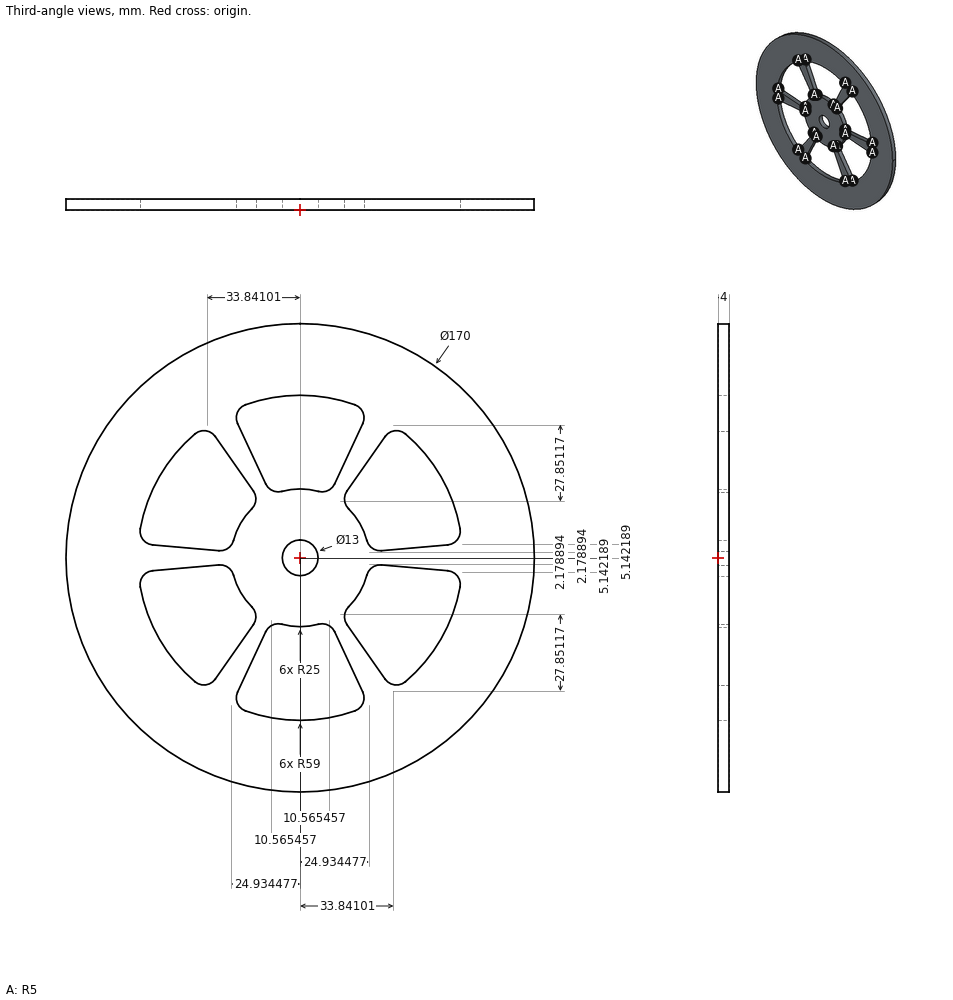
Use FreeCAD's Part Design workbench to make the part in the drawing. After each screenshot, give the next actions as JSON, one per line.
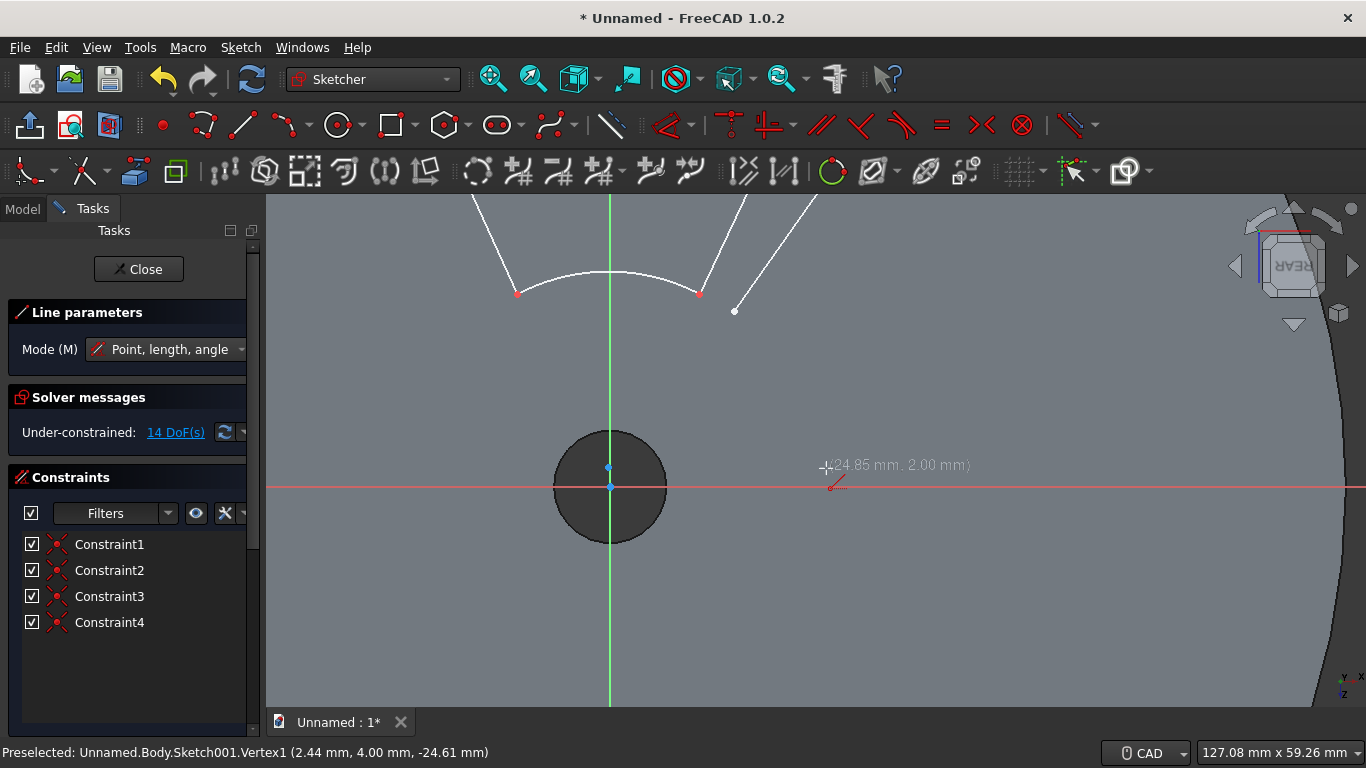
{"action": "left_click", "coordinate": [826, 468]}
{"action": "left_click", "coordinate": [1119, 442]}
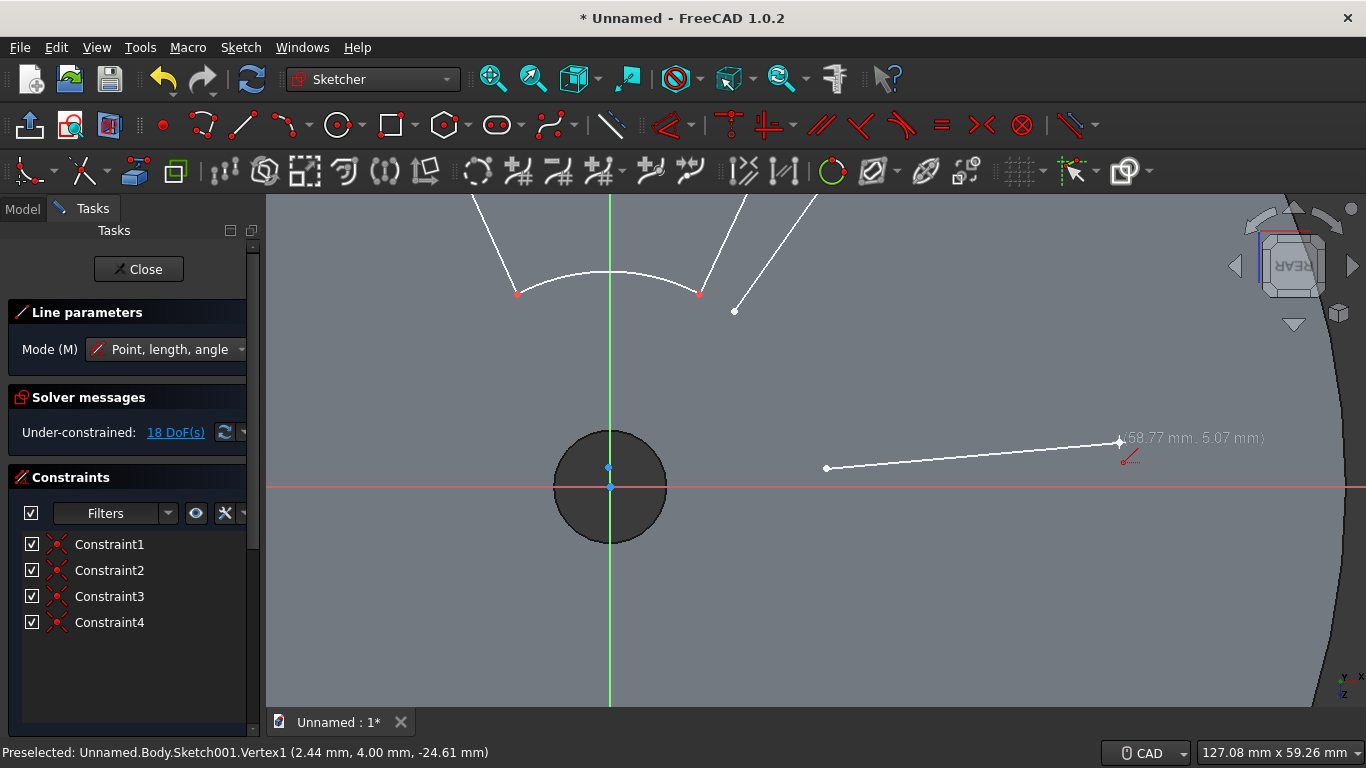
{"action": "left_click", "coordinate": [284, 126]}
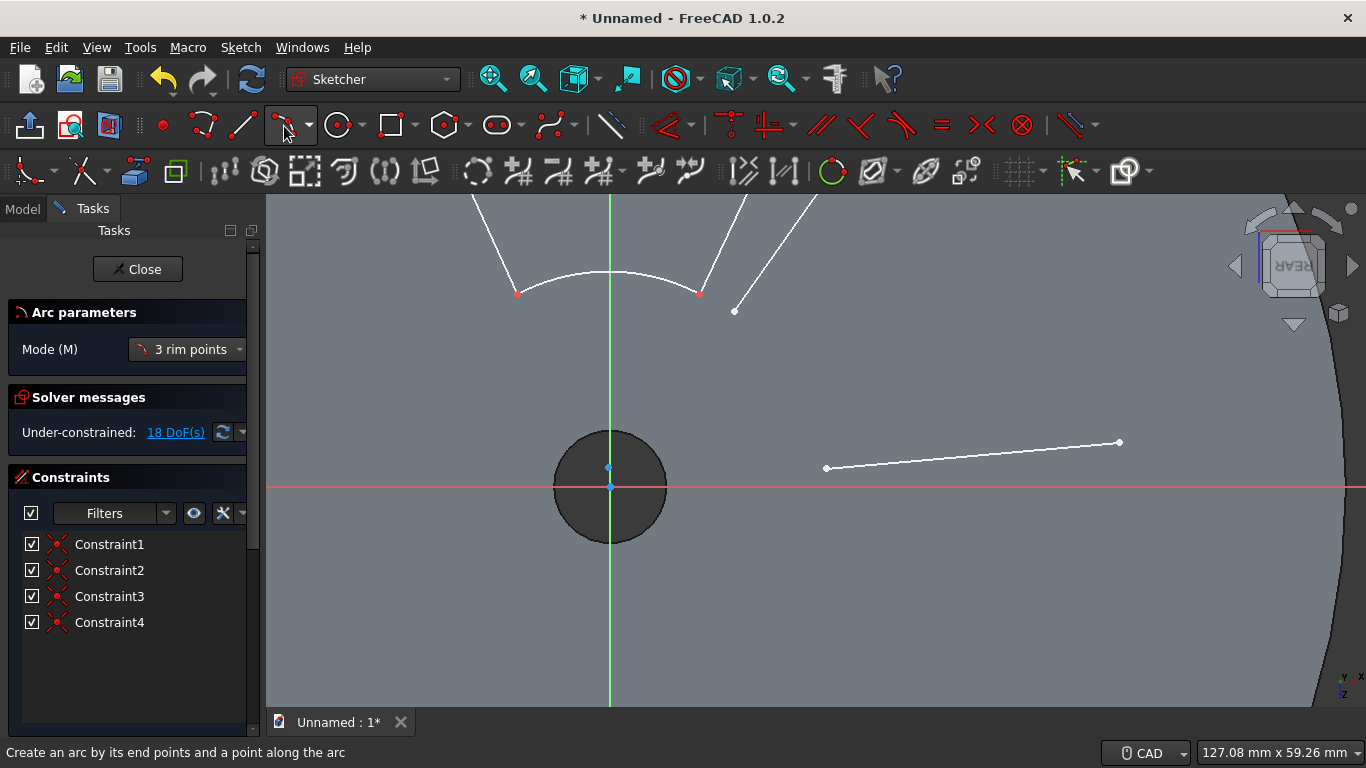
{"action": "left_click", "coordinate": [734, 312]}
{"action": "left_click", "coordinate": [826, 469]}
{"action": "left_click", "coordinate": [798, 379]}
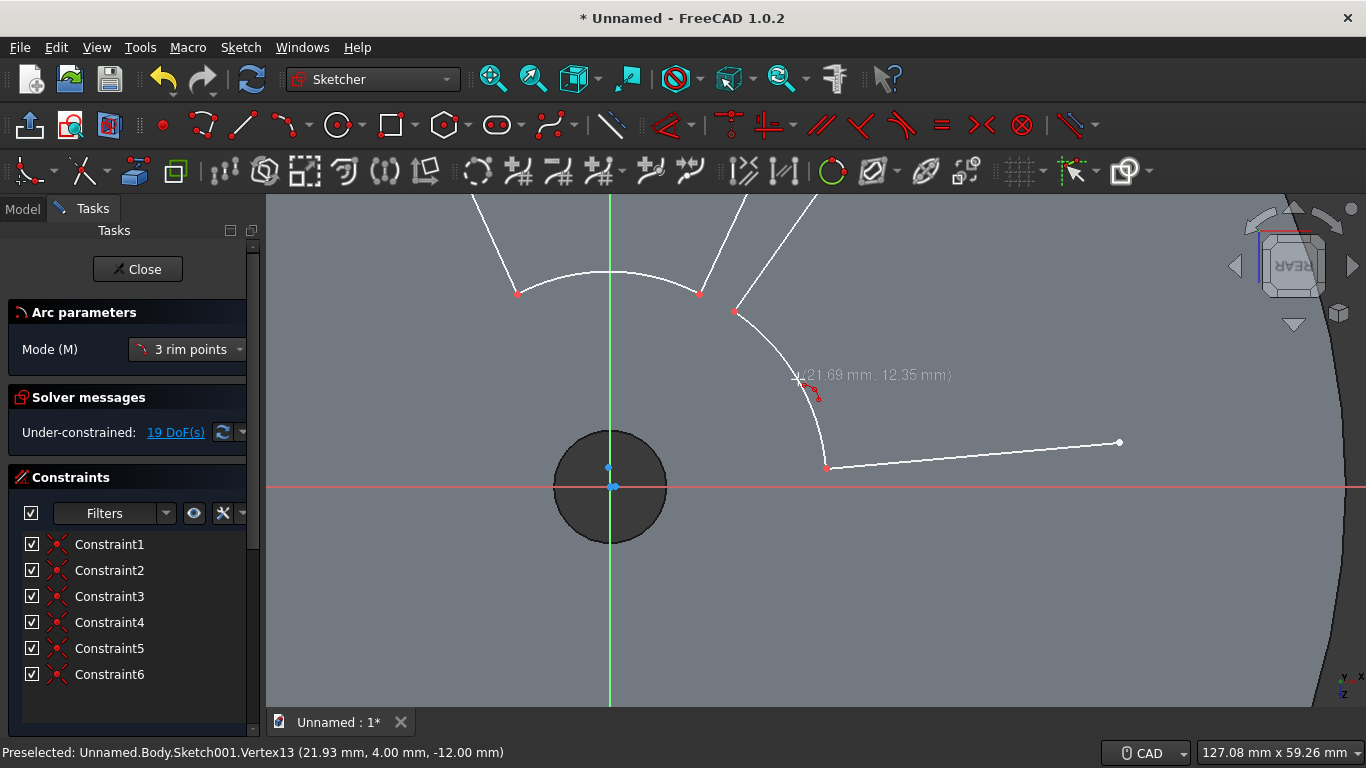
{"action": "left_click", "coordinate": [1119, 443]}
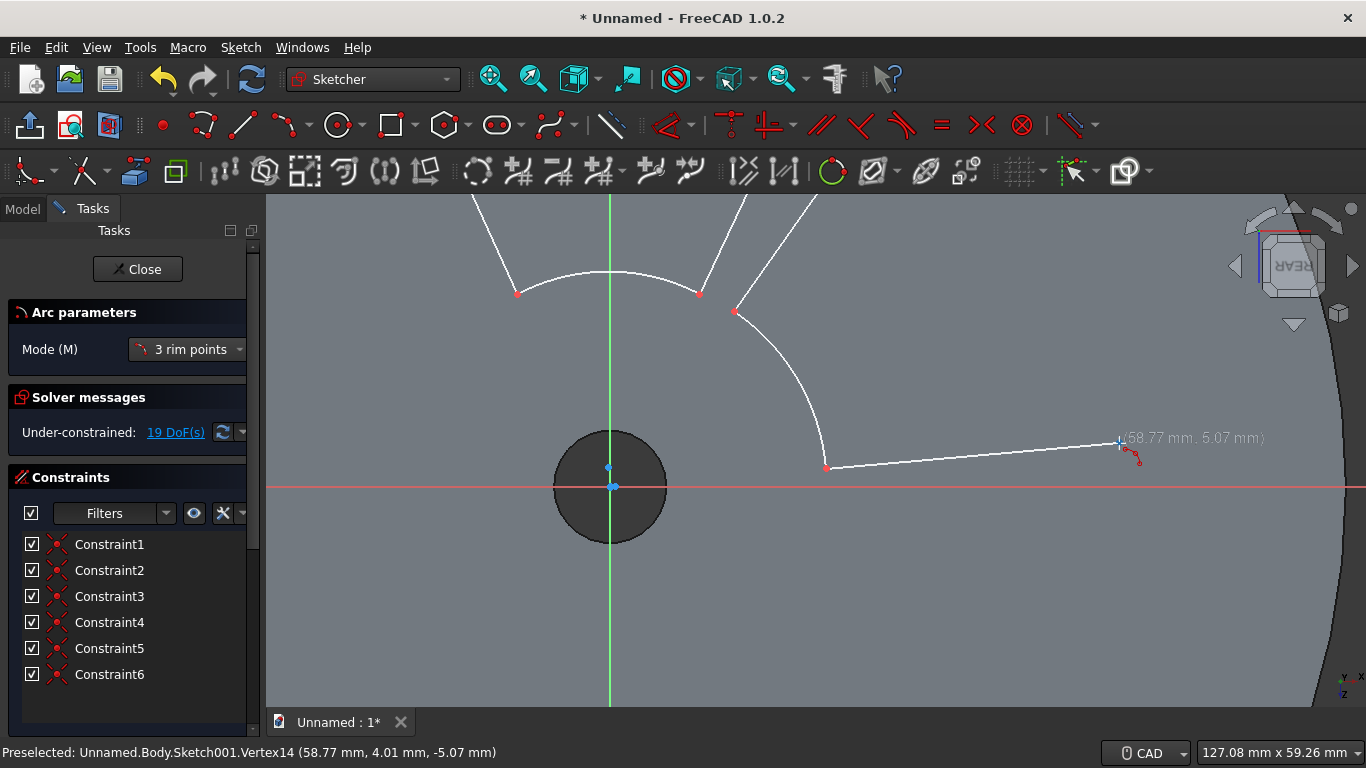
{"action": "scroll", "coordinate": [807, 435], "scroll_direction": "down", "scroll_amount": 6}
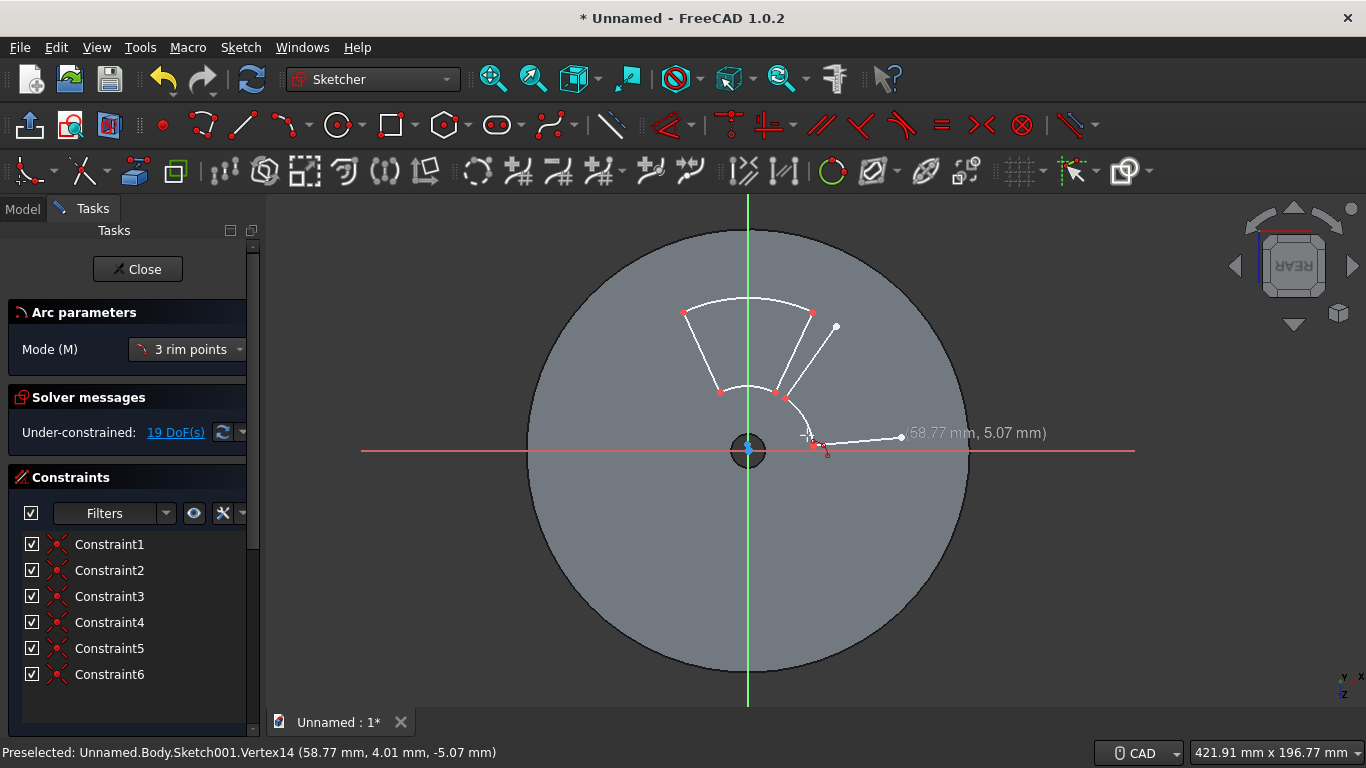
{"action": "left_click", "coordinate": [836, 326]}
{"action": "left_click", "coordinate": [881, 374]}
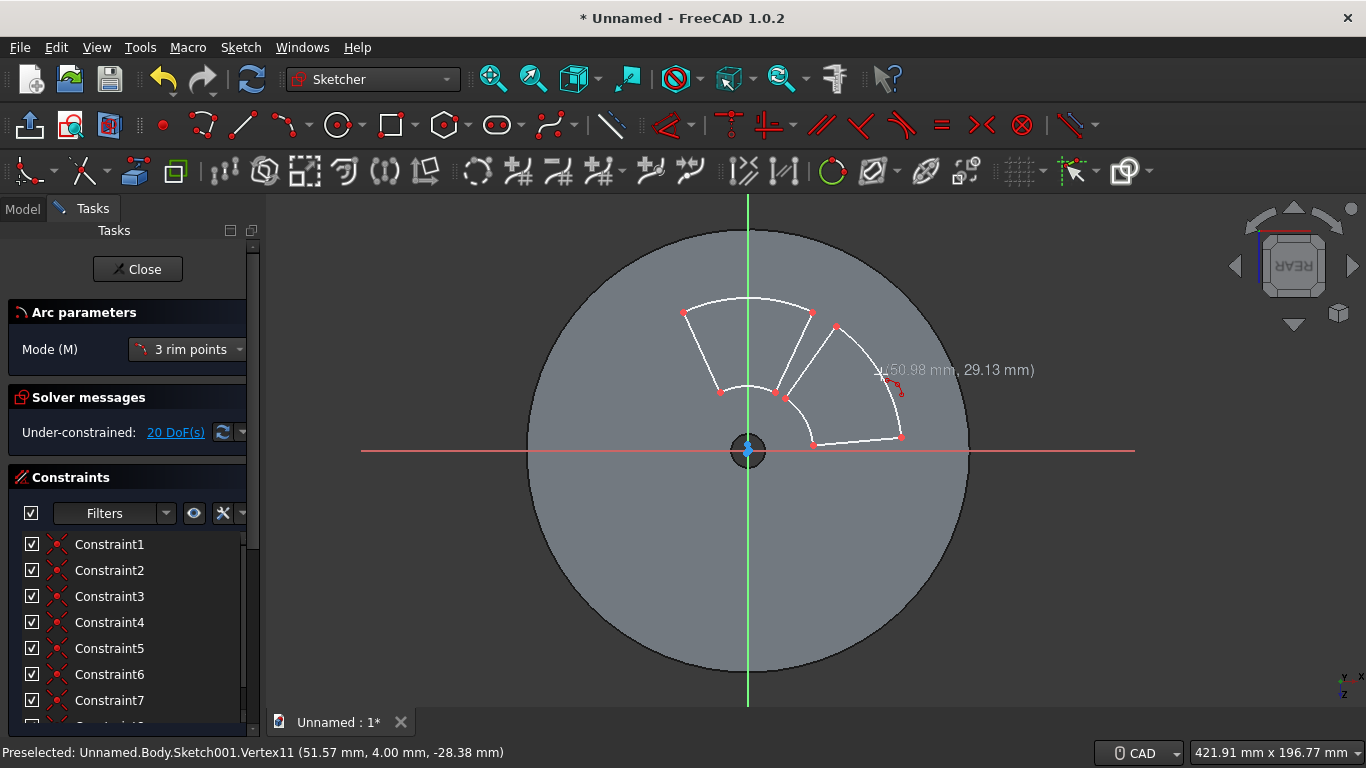
{"action": "left_click", "coordinate": [244, 126]}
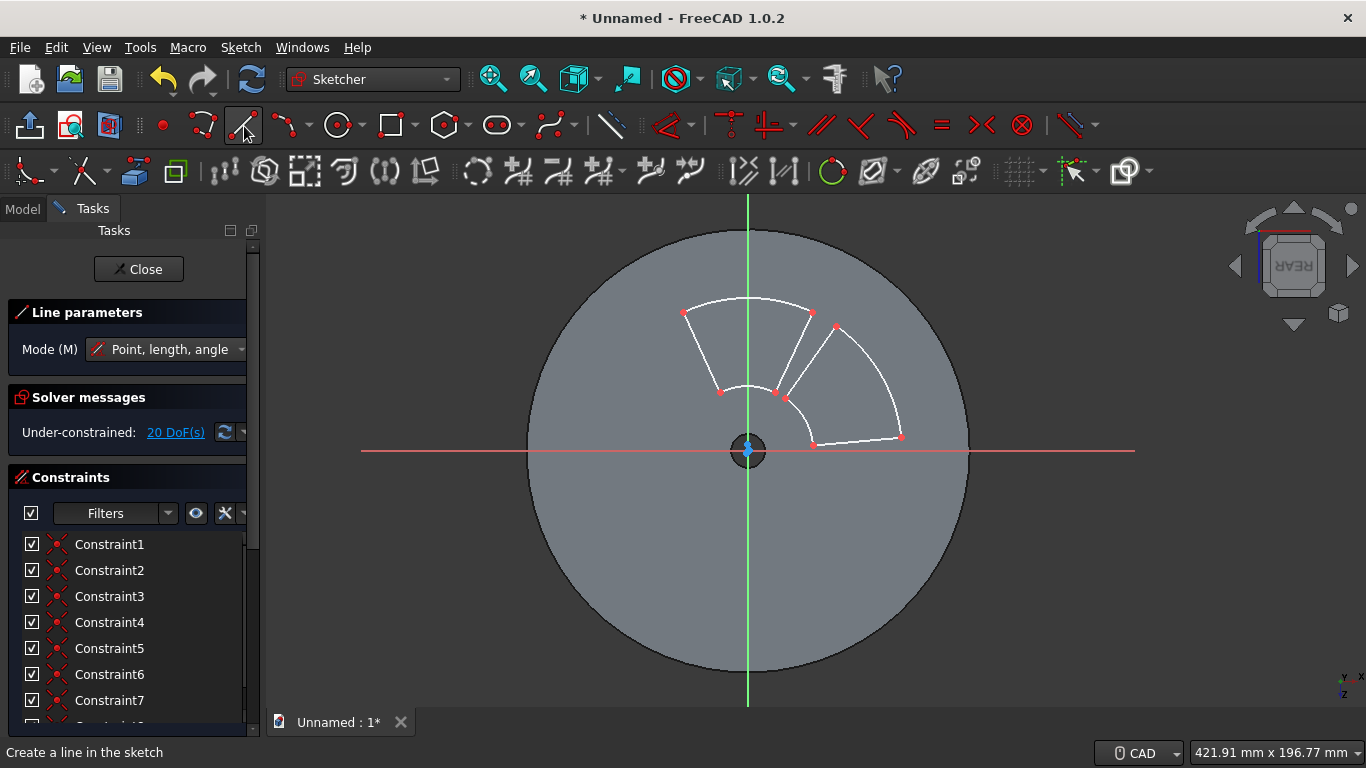
{"action": "left_click", "coordinate": [901, 464]}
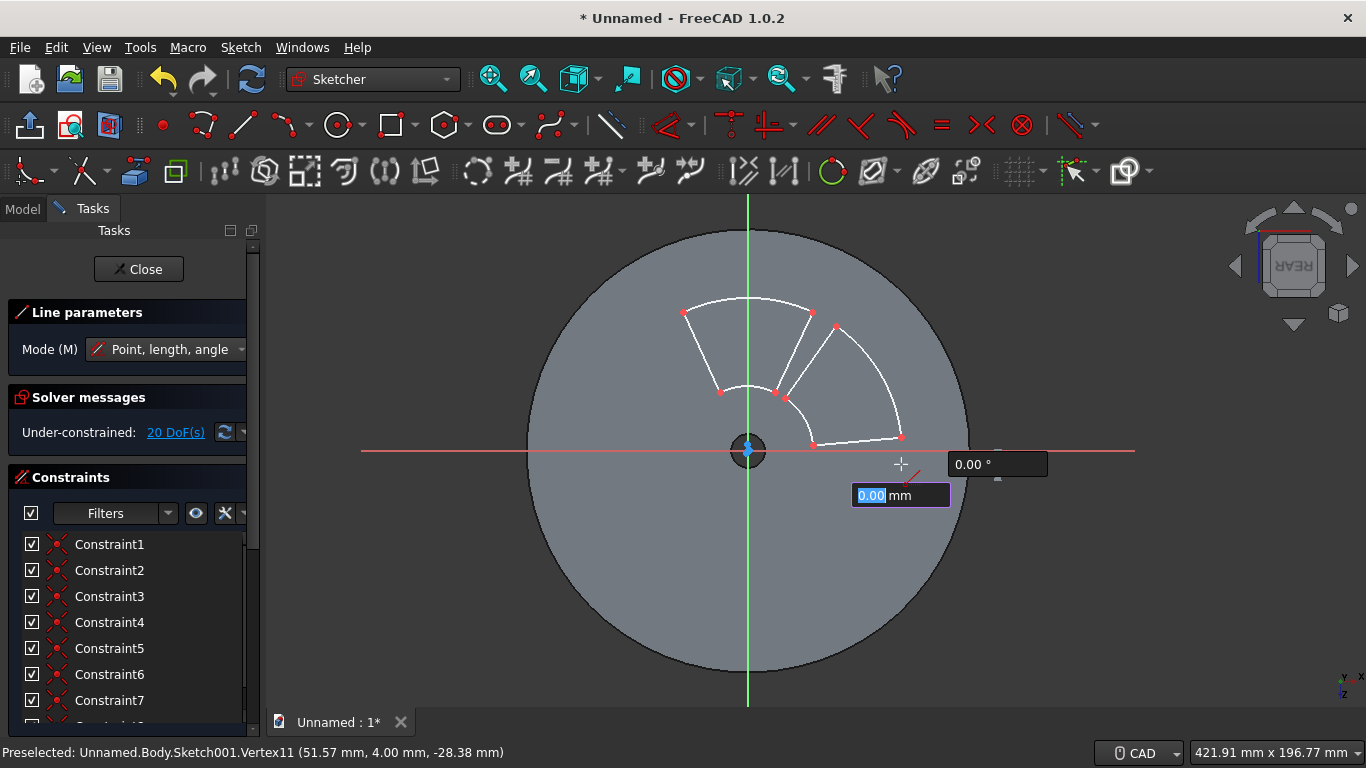
{"action": "scroll", "coordinate": [813, 457], "scroll_direction": "up", "scroll_amount": 6}